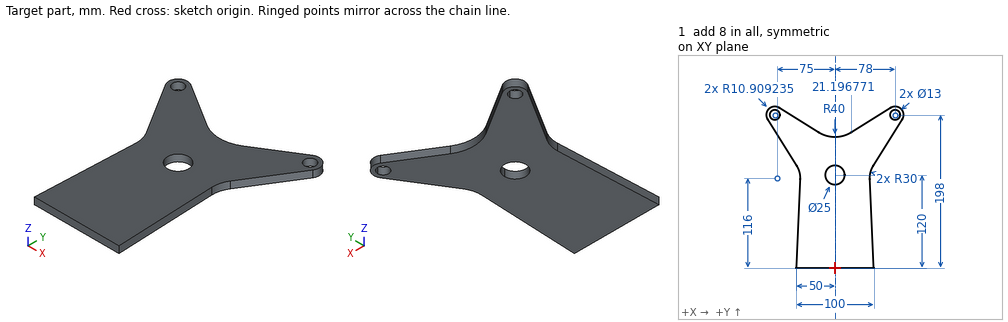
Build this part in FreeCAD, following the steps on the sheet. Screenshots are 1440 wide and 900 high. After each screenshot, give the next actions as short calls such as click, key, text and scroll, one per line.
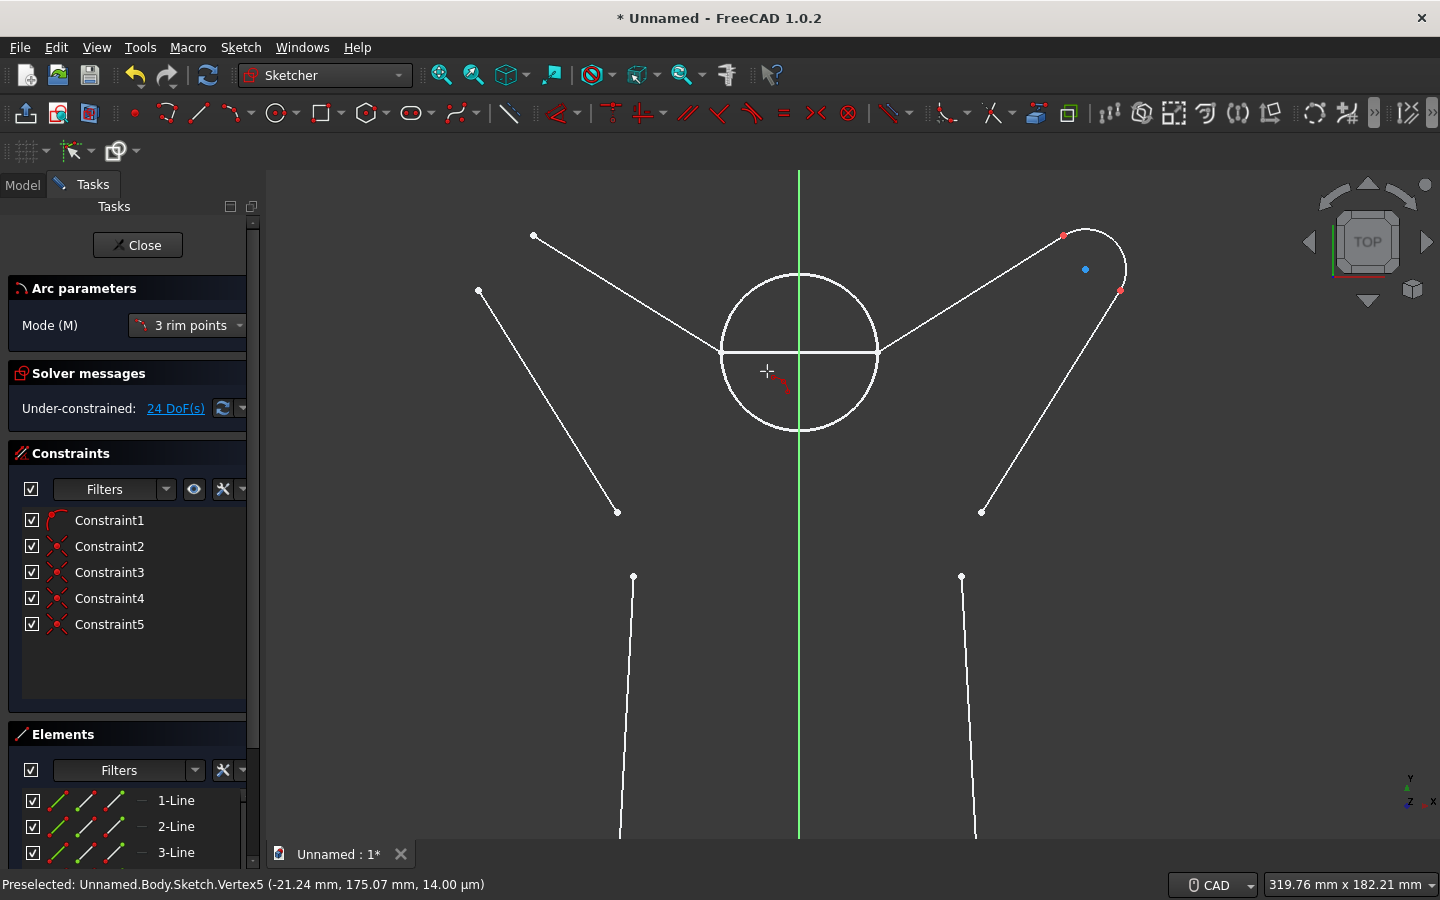
click(767, 370)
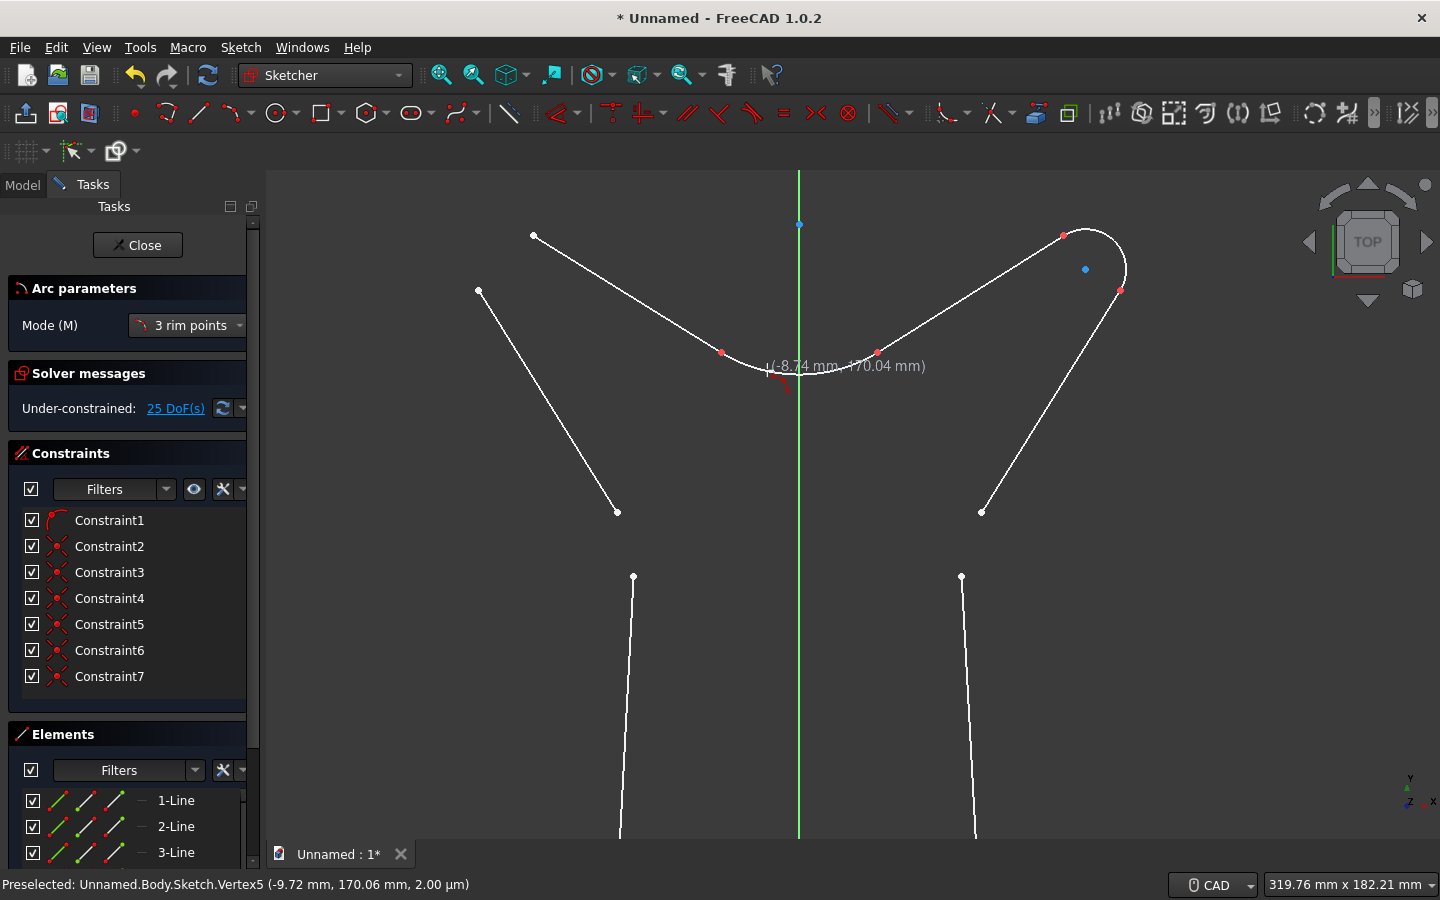
click(533, 236)
click(479, 291)
click(484, 240)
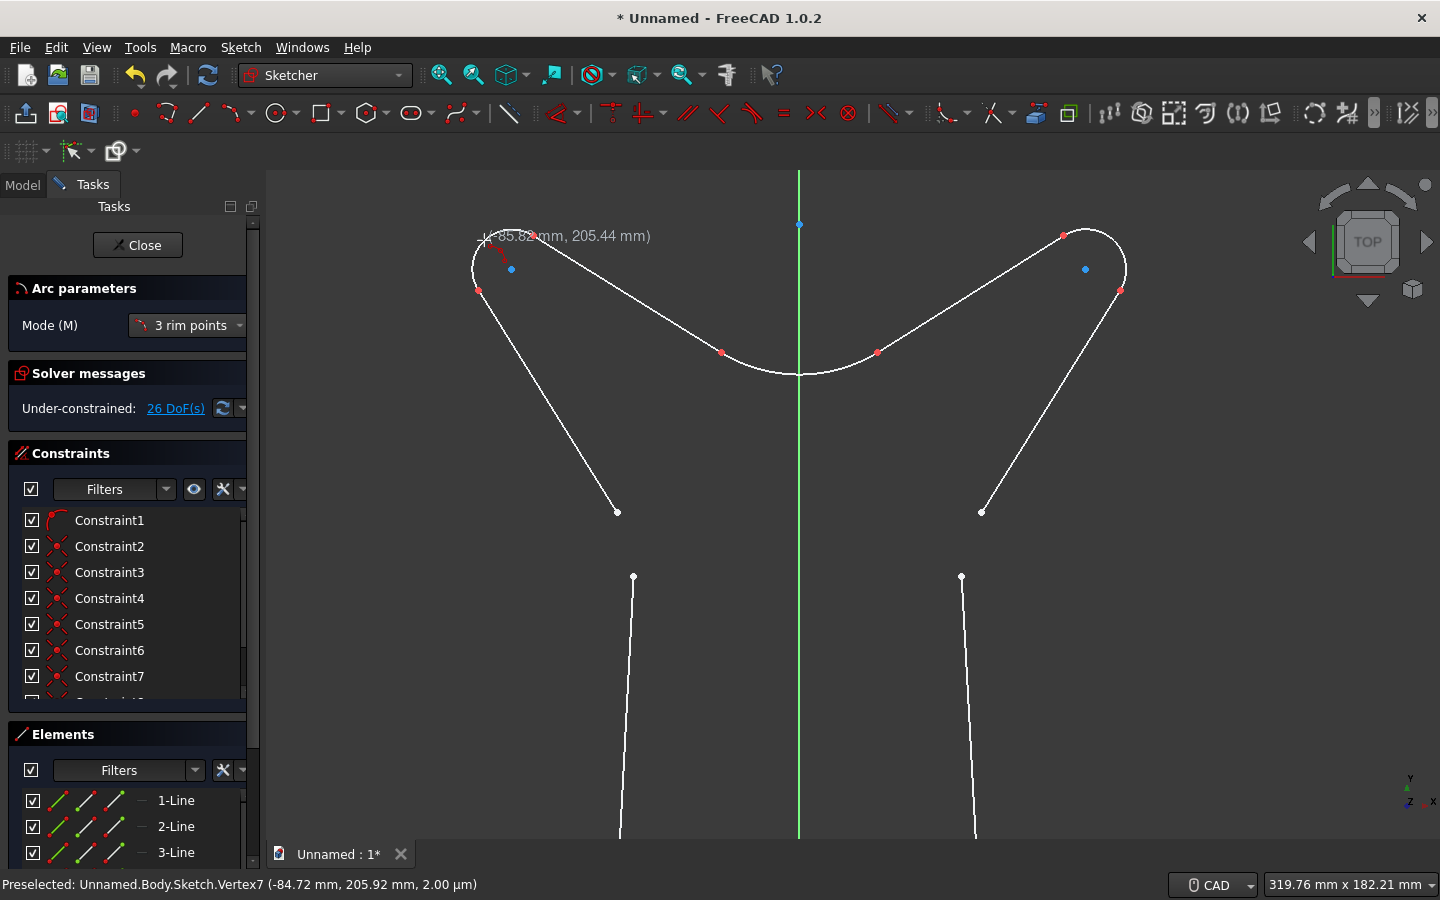
click(617, 513)
click(634, 577)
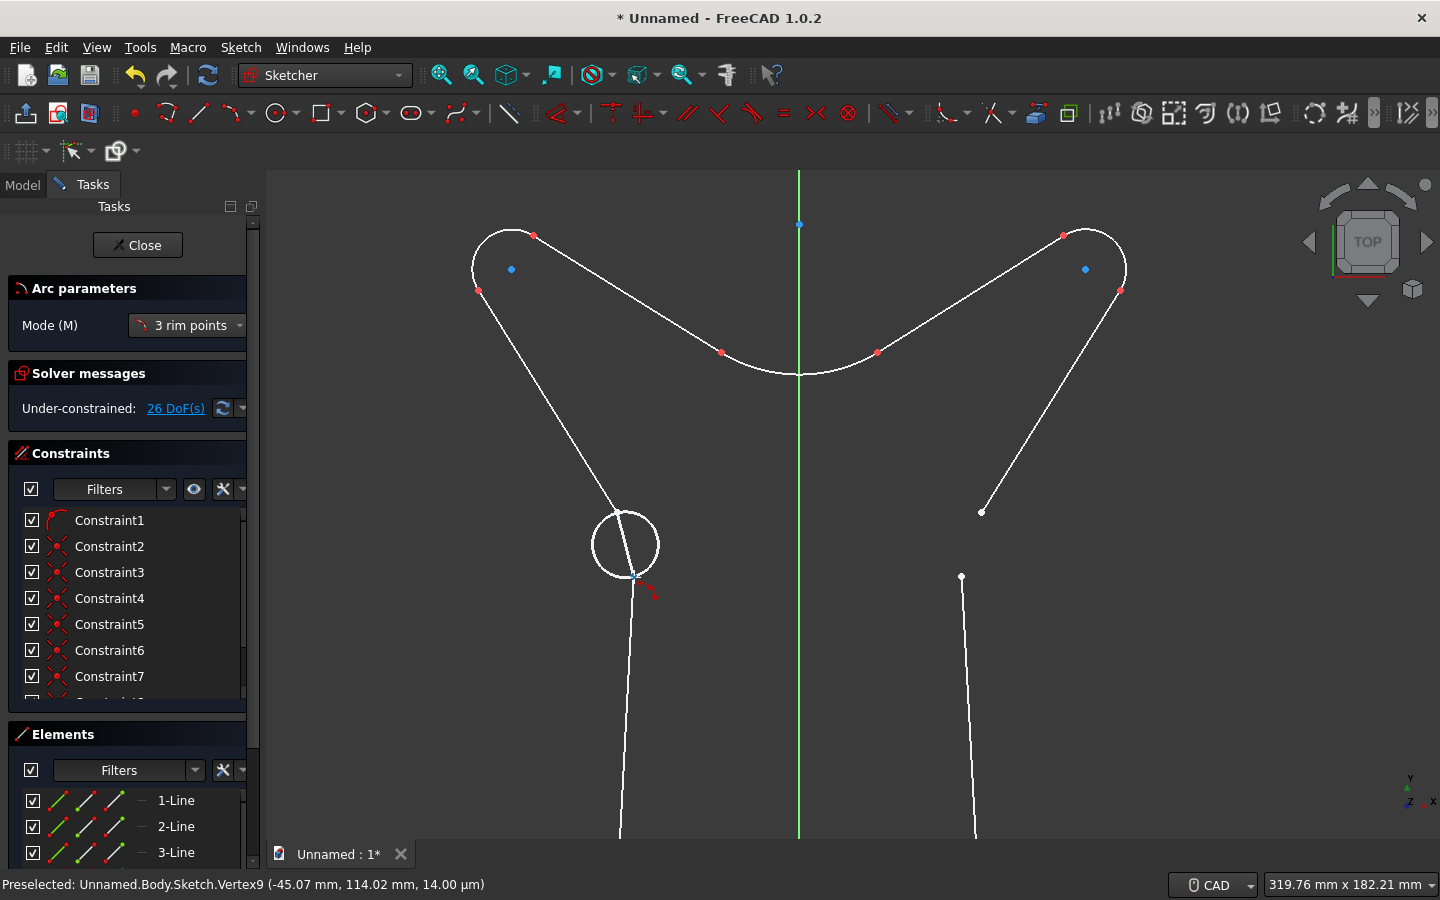
scroll(630, 541, up, 6)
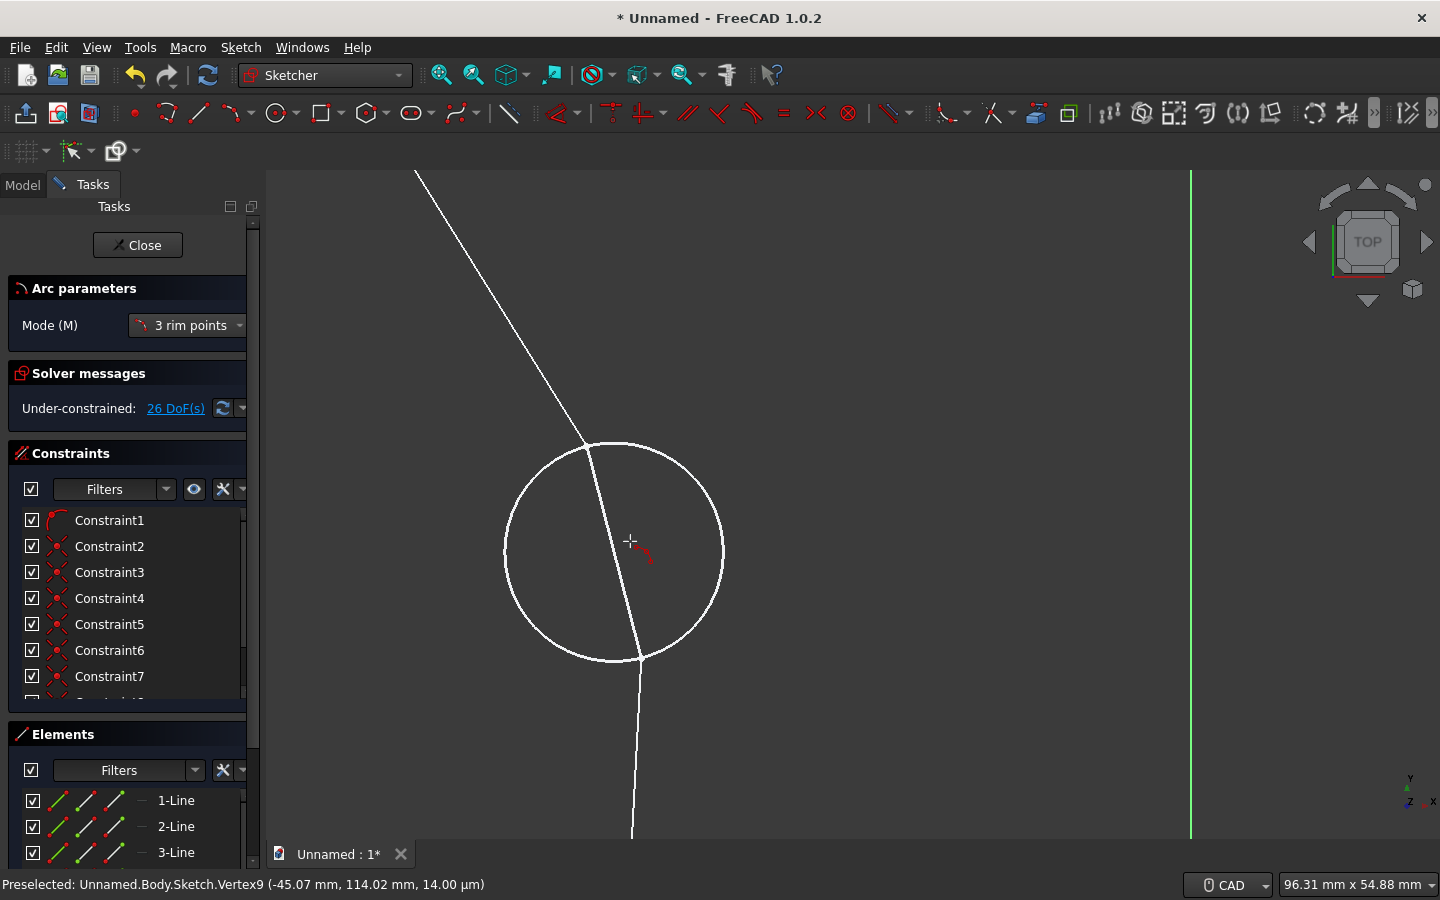
click(630, 541)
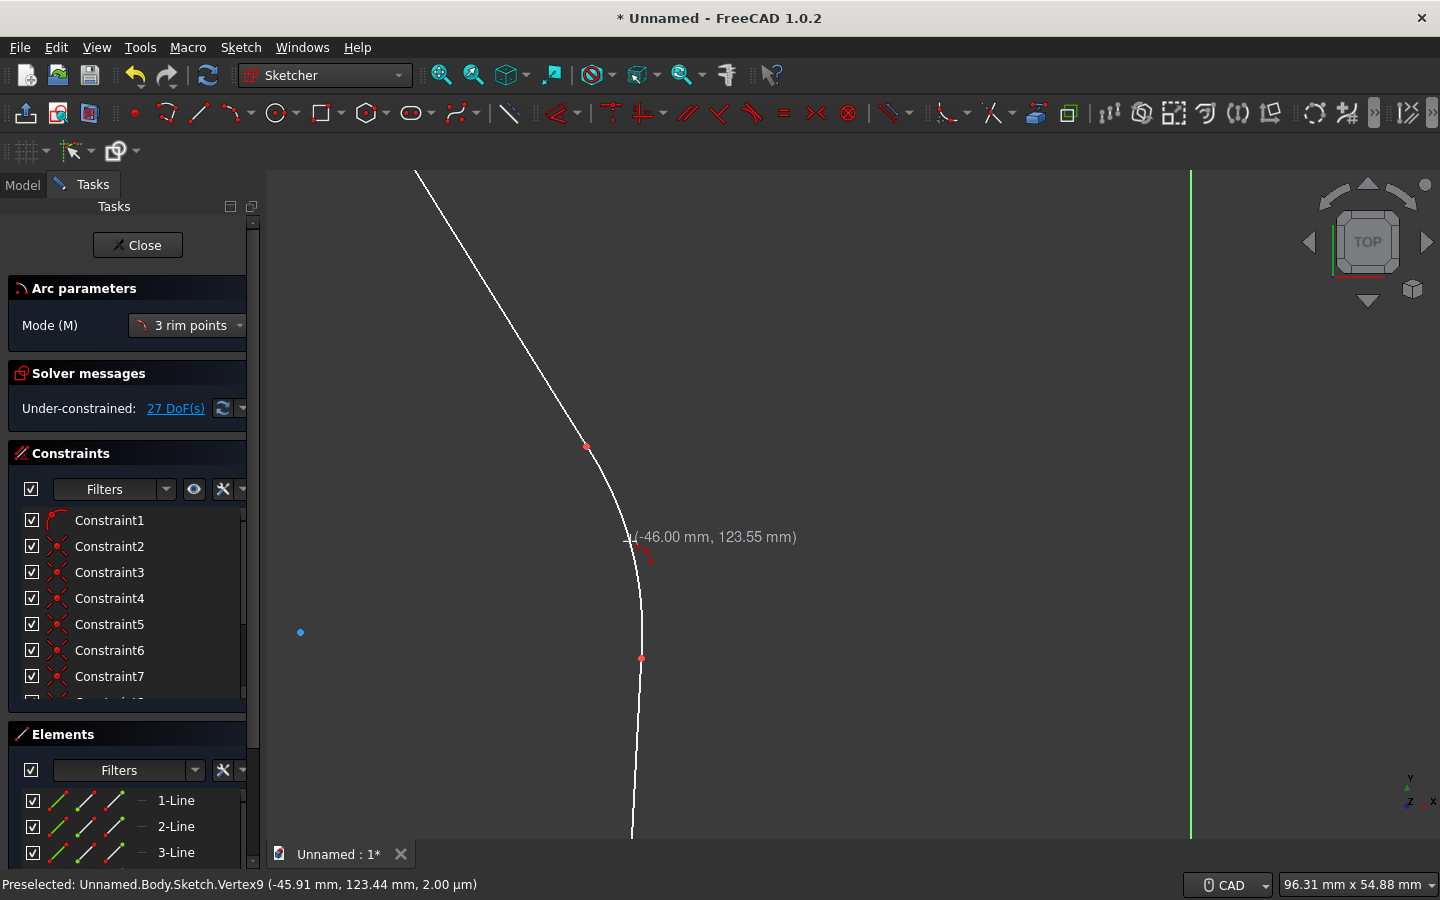
scroll(704, 449, down, 9)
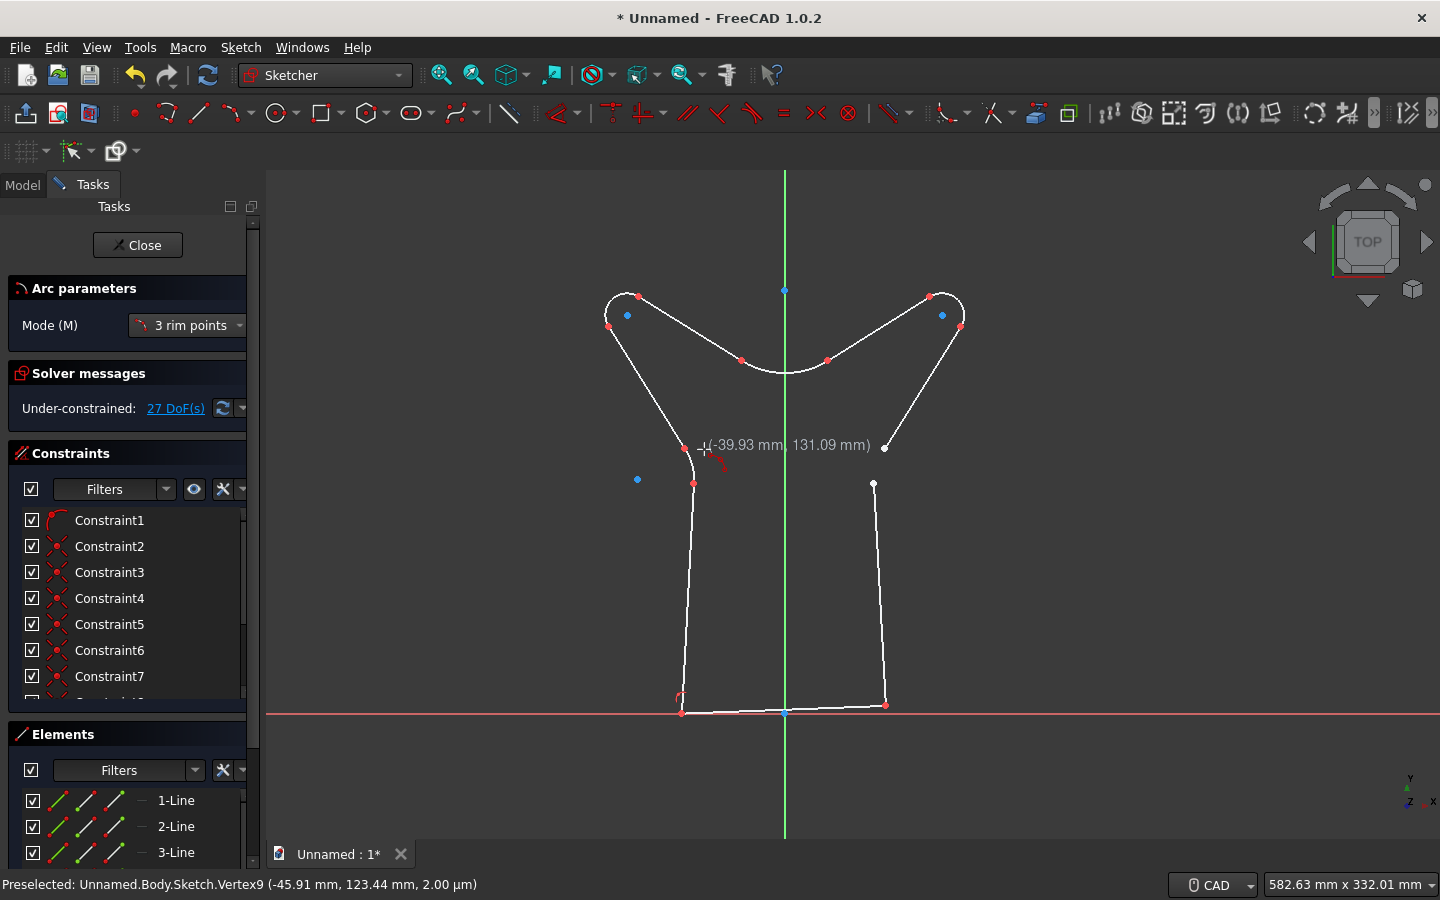
click(874, 484)
click(885, 449)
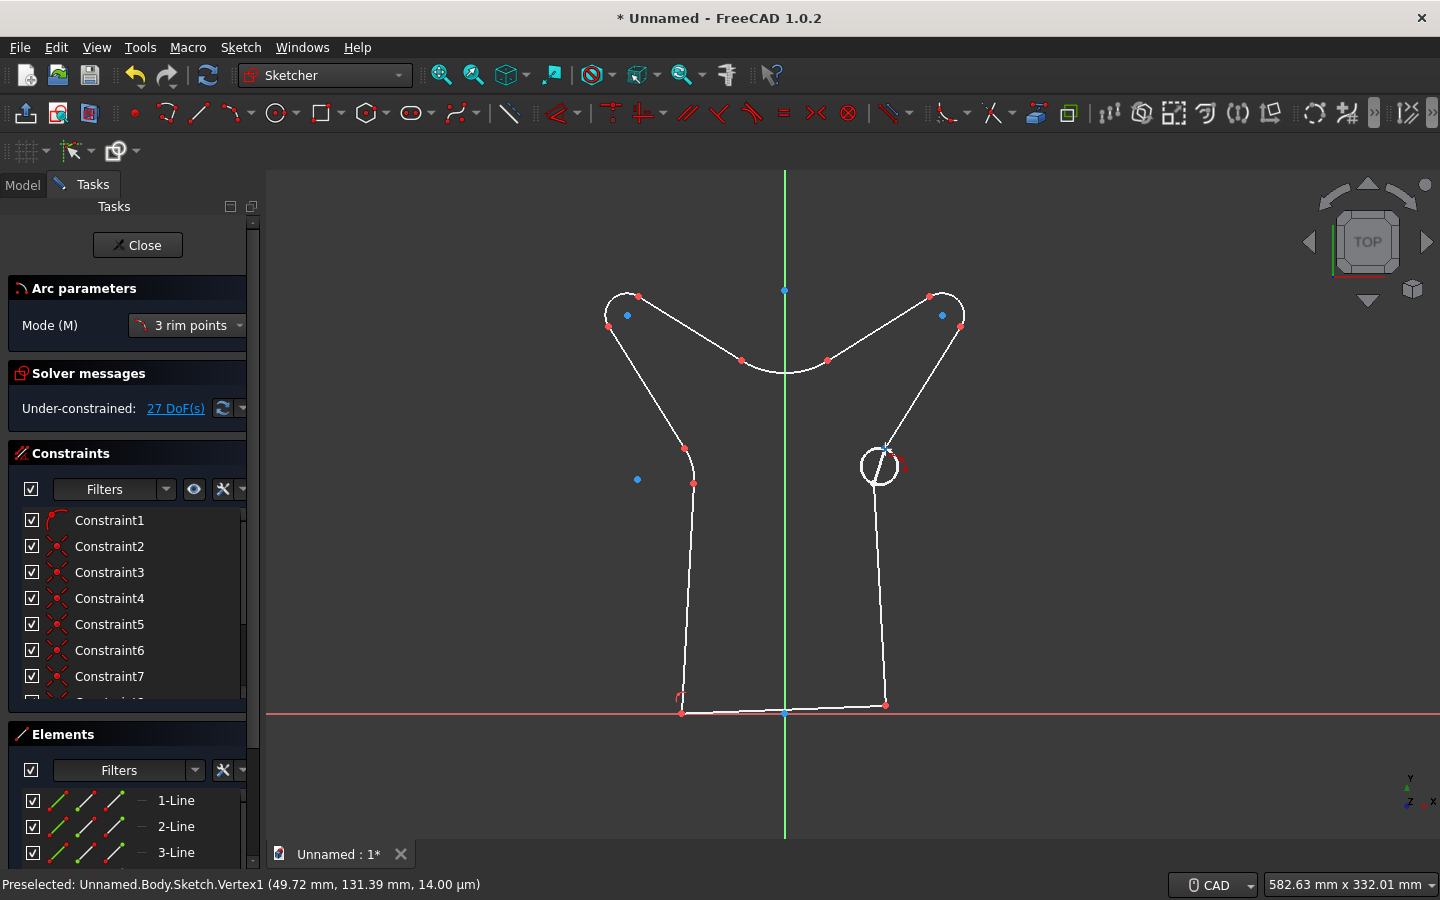
scroll(877, 465, up, 9)